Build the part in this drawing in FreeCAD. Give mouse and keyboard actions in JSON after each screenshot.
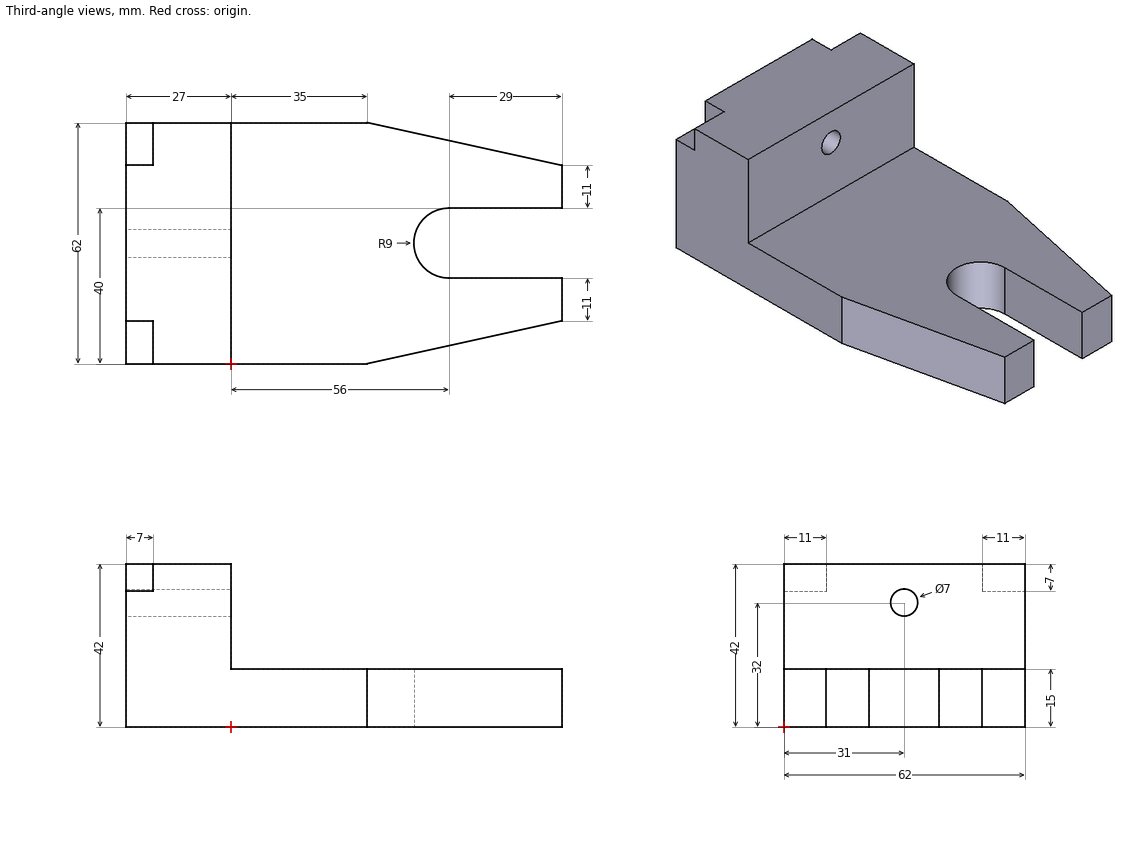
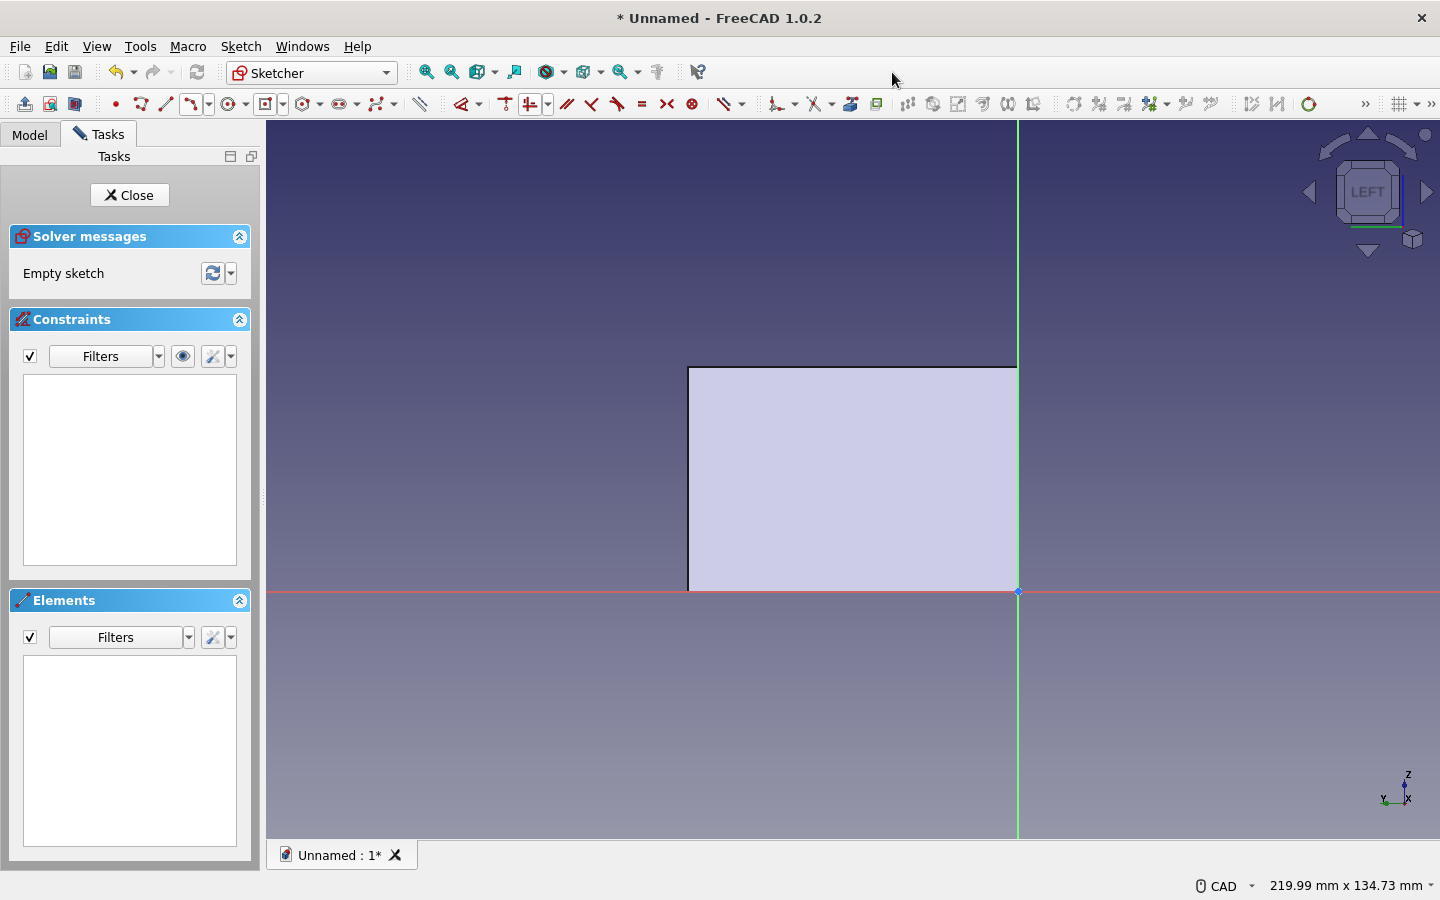
{"action": "scroll", "coordinate": [909, 480], "scroll_direction": "up", "scroll_amount": 4}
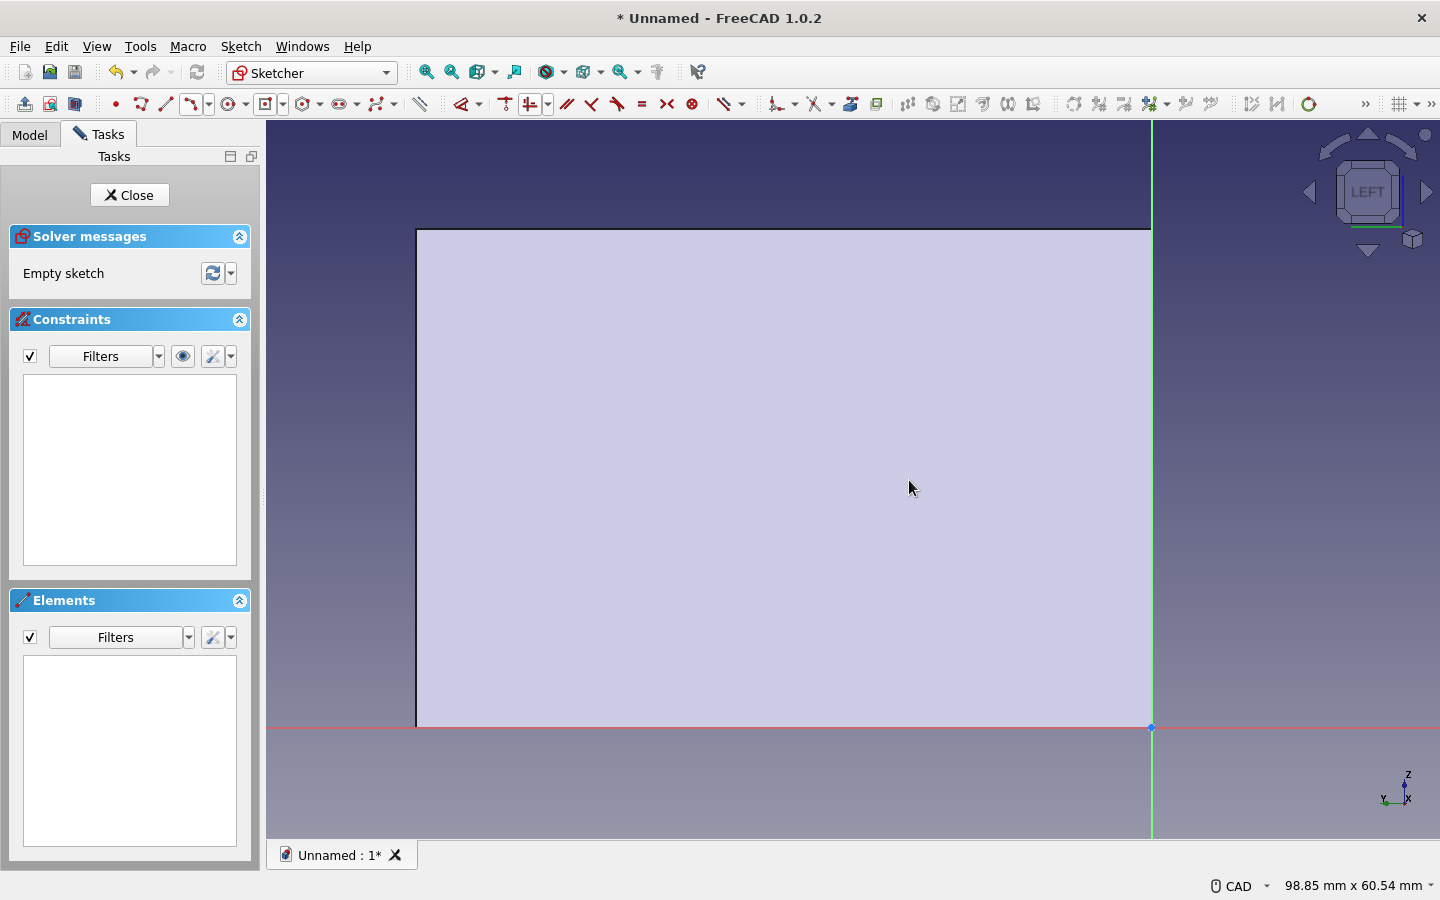
{"action": "key", "text": "g r"}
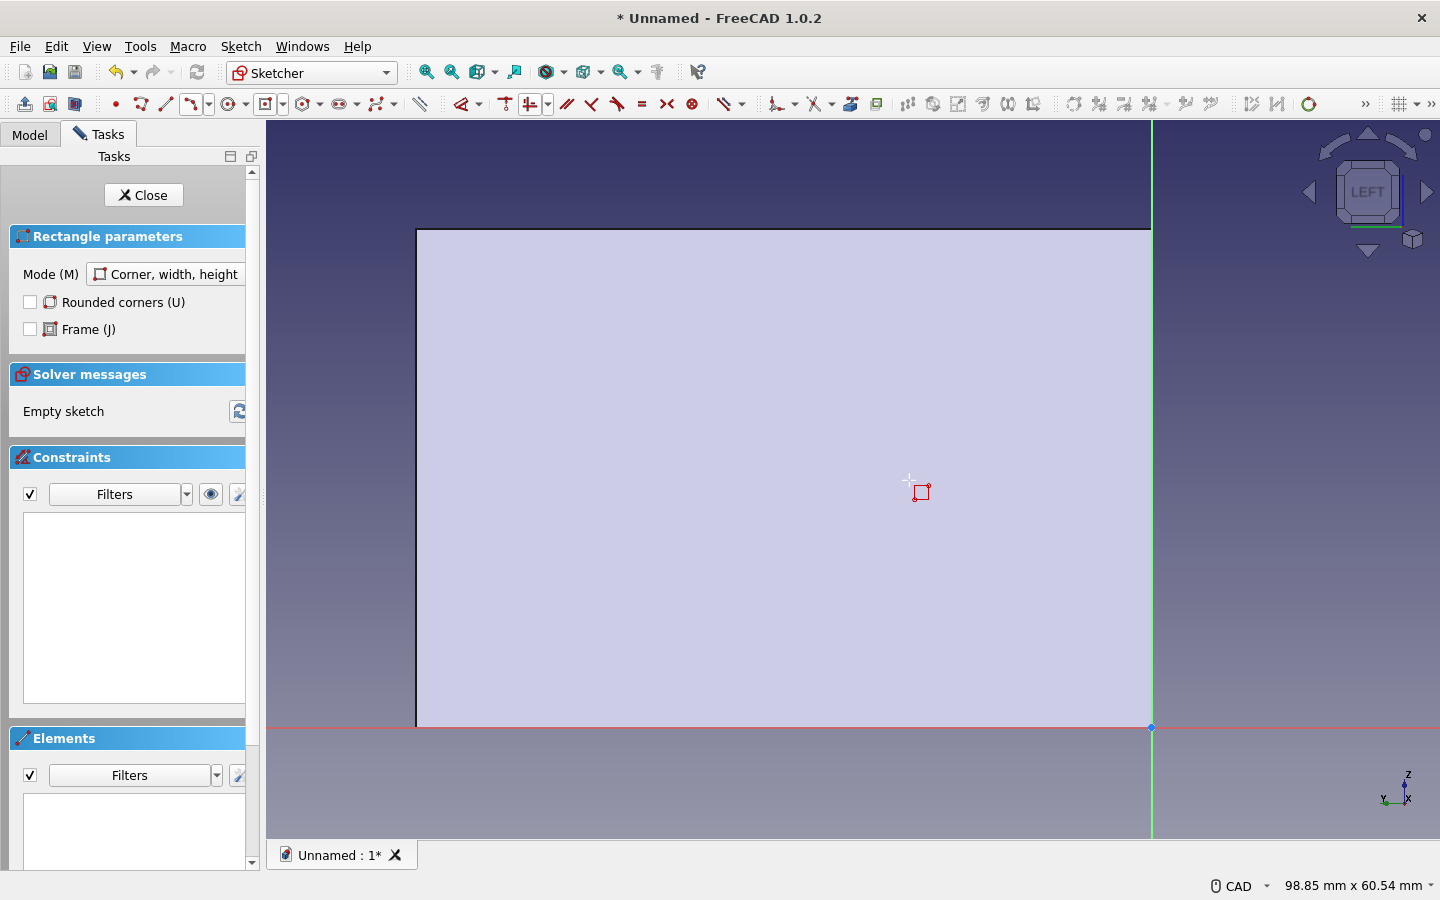
{"action": "left_click", "coordinate": [416, 229]}
{"action": "left_click", "coordinate": [546, 312]}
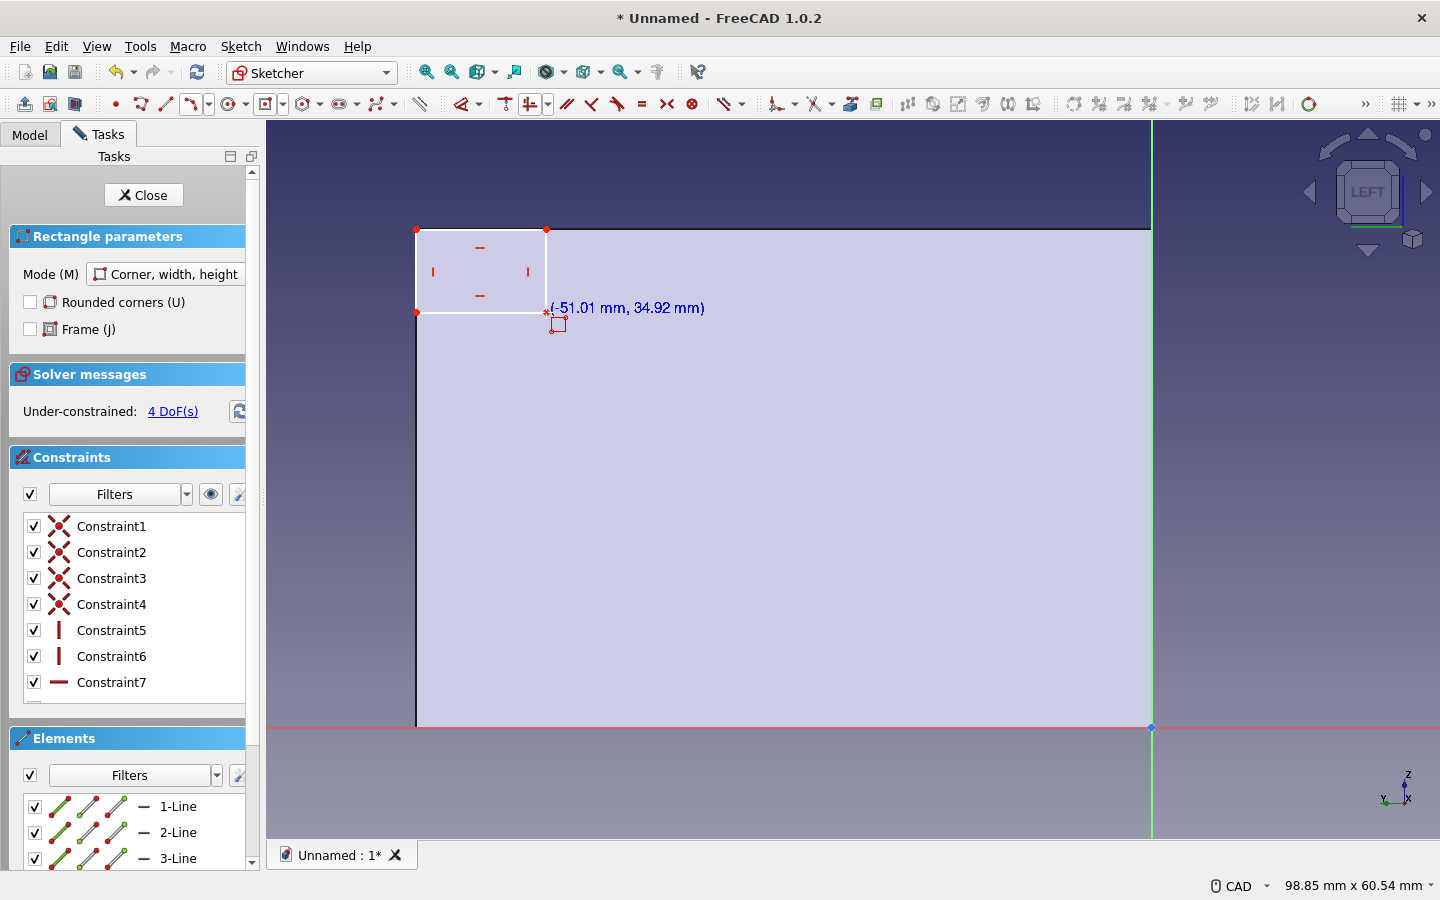
{"action": "left_click", "coordinate": [1021, 229]}
{"action": "left_click", "coordinate": [1152, 312]}
{"action": "key", "text": "Escape"}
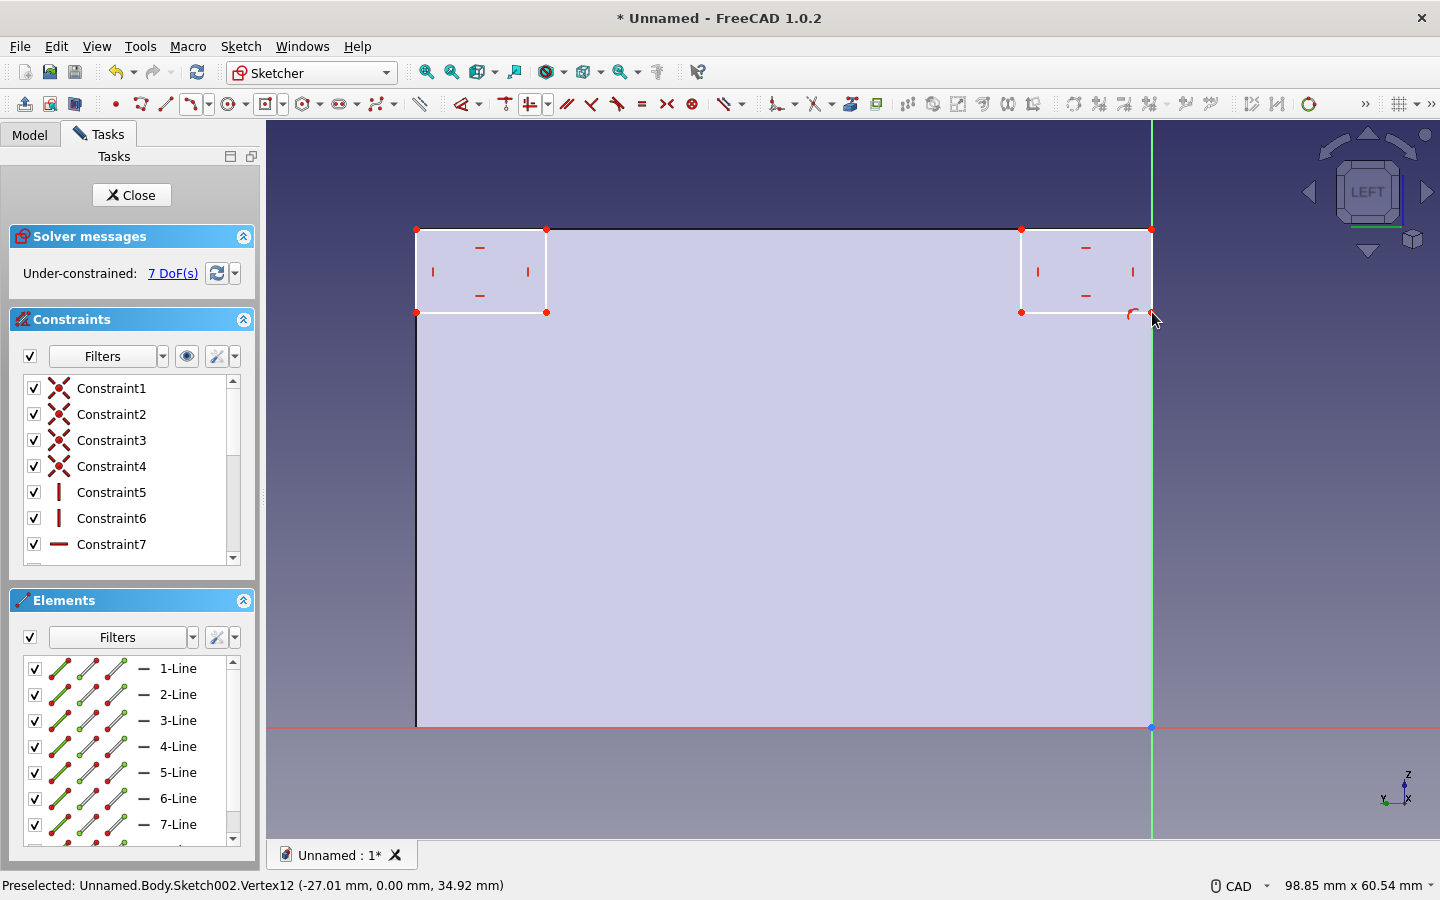
{"action": "left_click", "coordinate": [460, 104]}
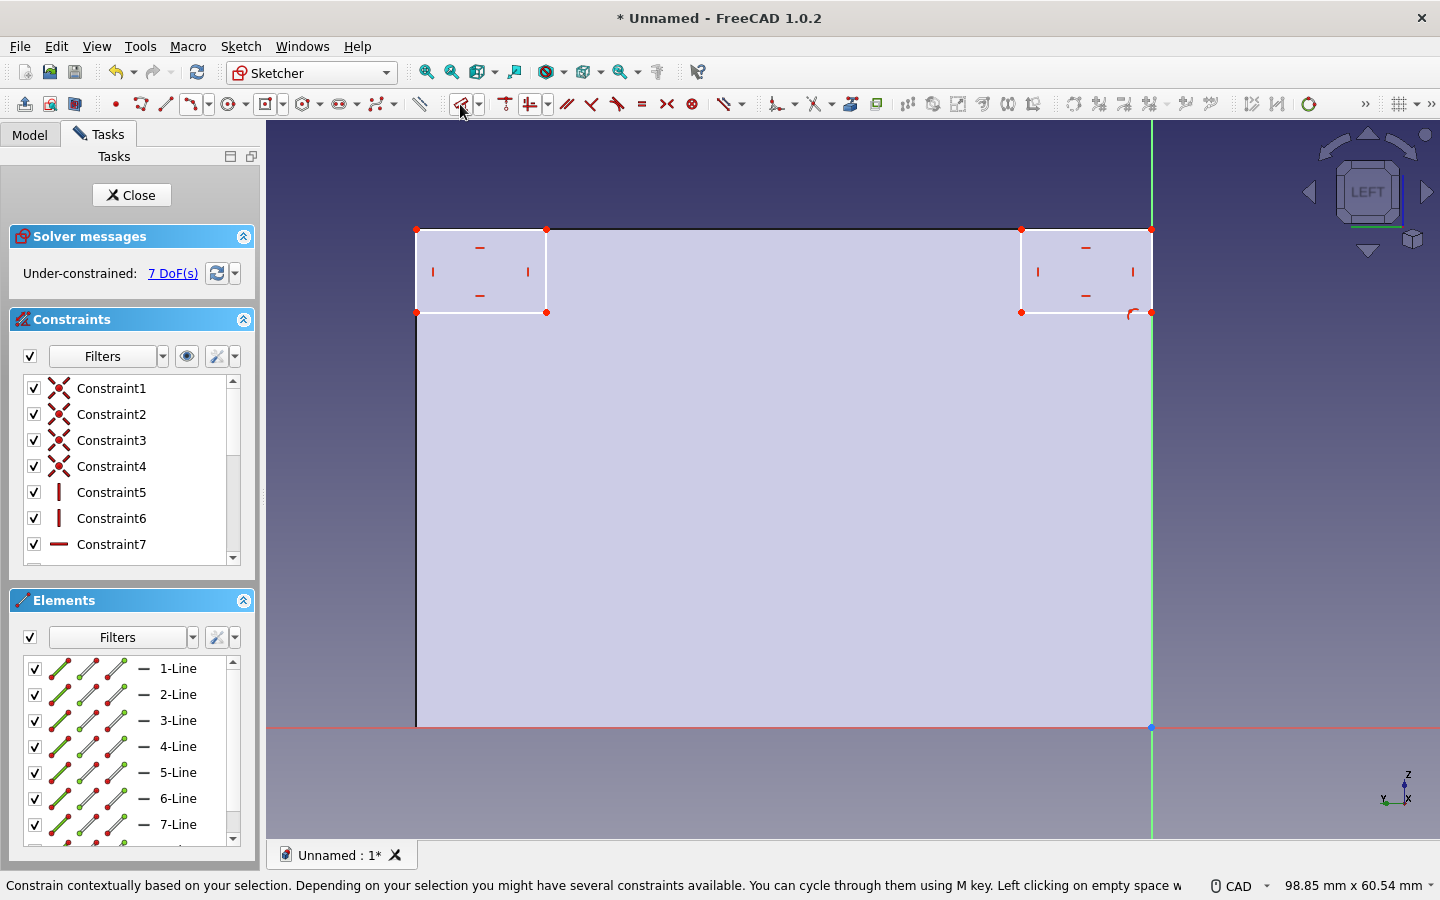
{"action": "left_click", "coordinate": [416, 255]}
{"action": "left_click", "coordinate": [382, 272]}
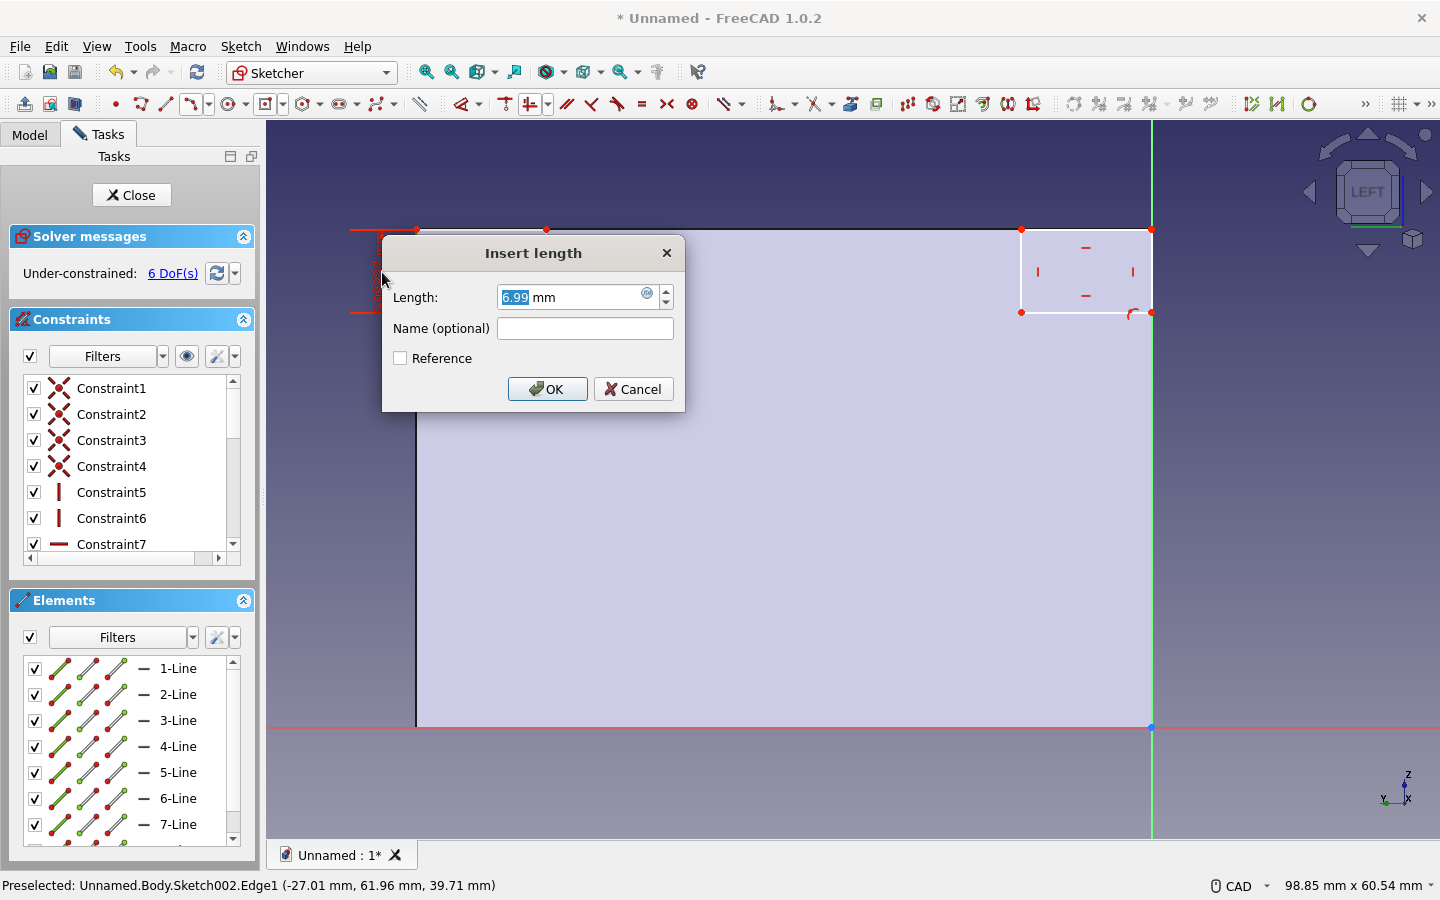
{"action": "type", "text": "7"}
{"action": "key", "text": "Return"}